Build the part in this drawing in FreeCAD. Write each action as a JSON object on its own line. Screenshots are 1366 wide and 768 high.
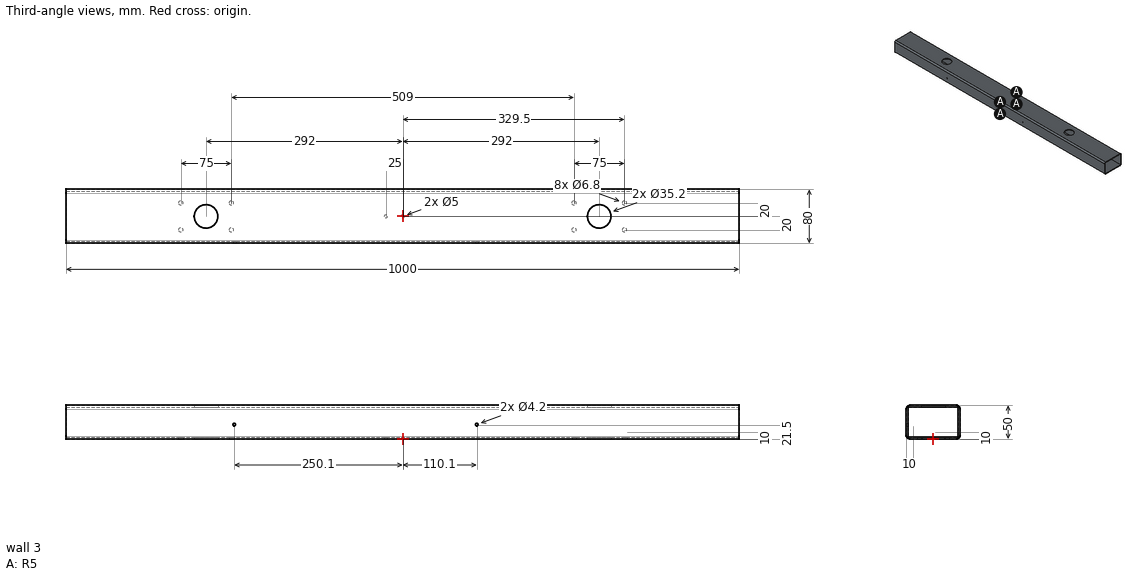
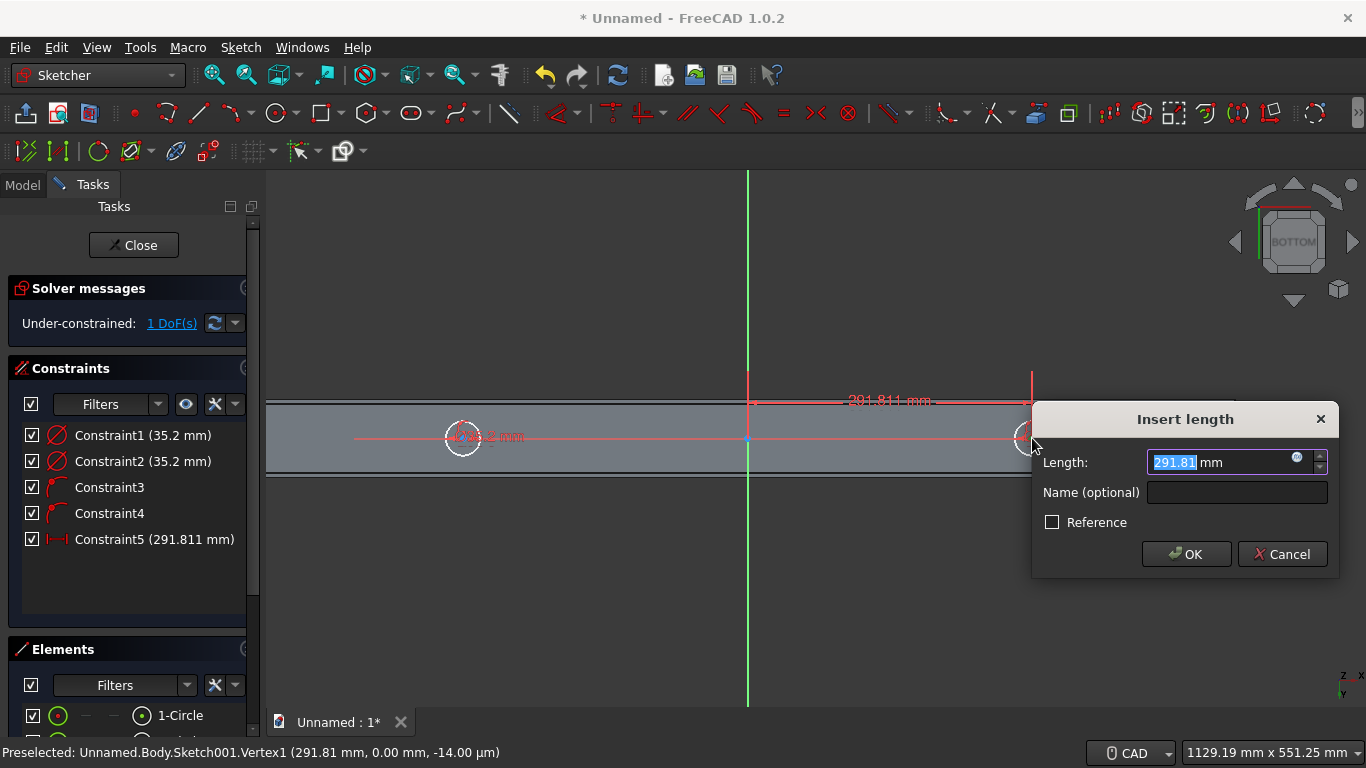
{"action": "type", "text": "292"}
{"action": "key", "text": "Return"}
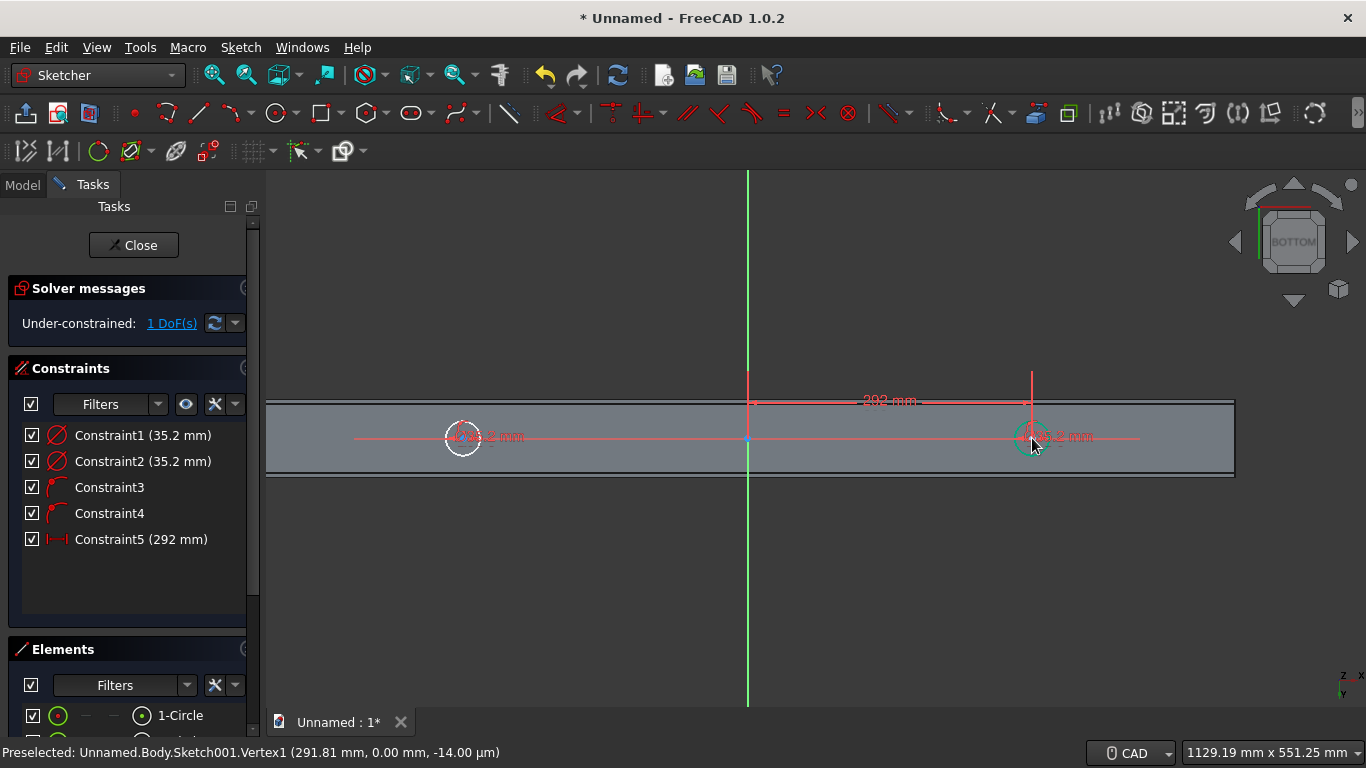
{"action": "left_click", "coordinate": [463, 438]}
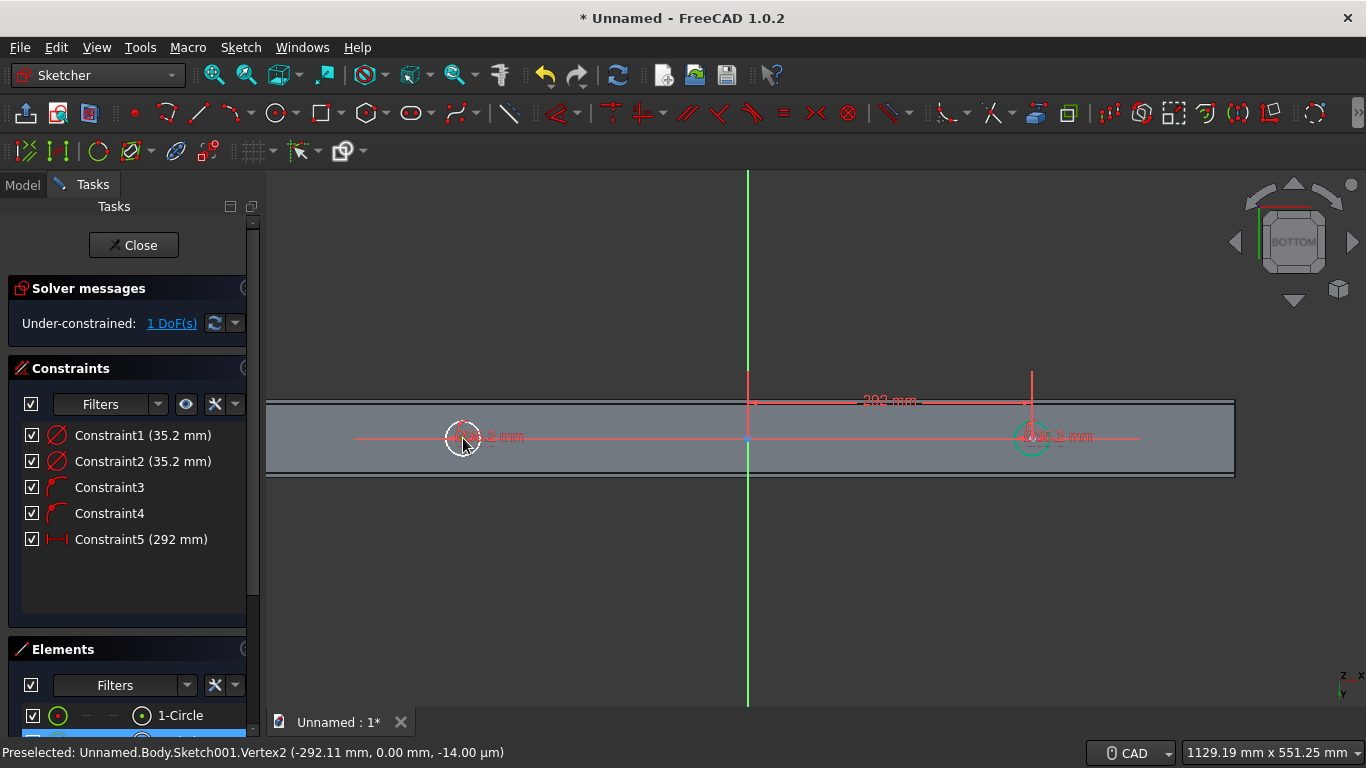
{"action": "key", "text": "l"}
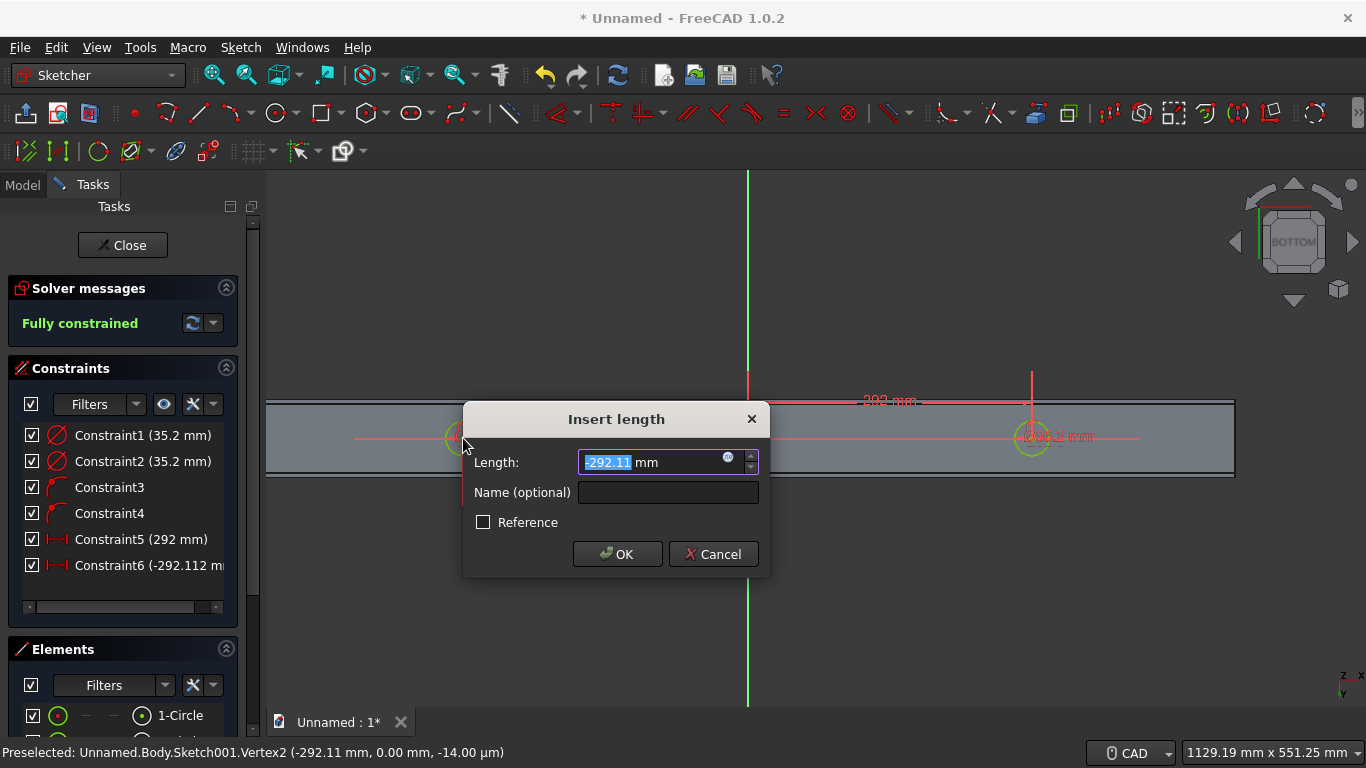
{"action": "type", "text": "-292"}
{"action": "key", "text": "Return"}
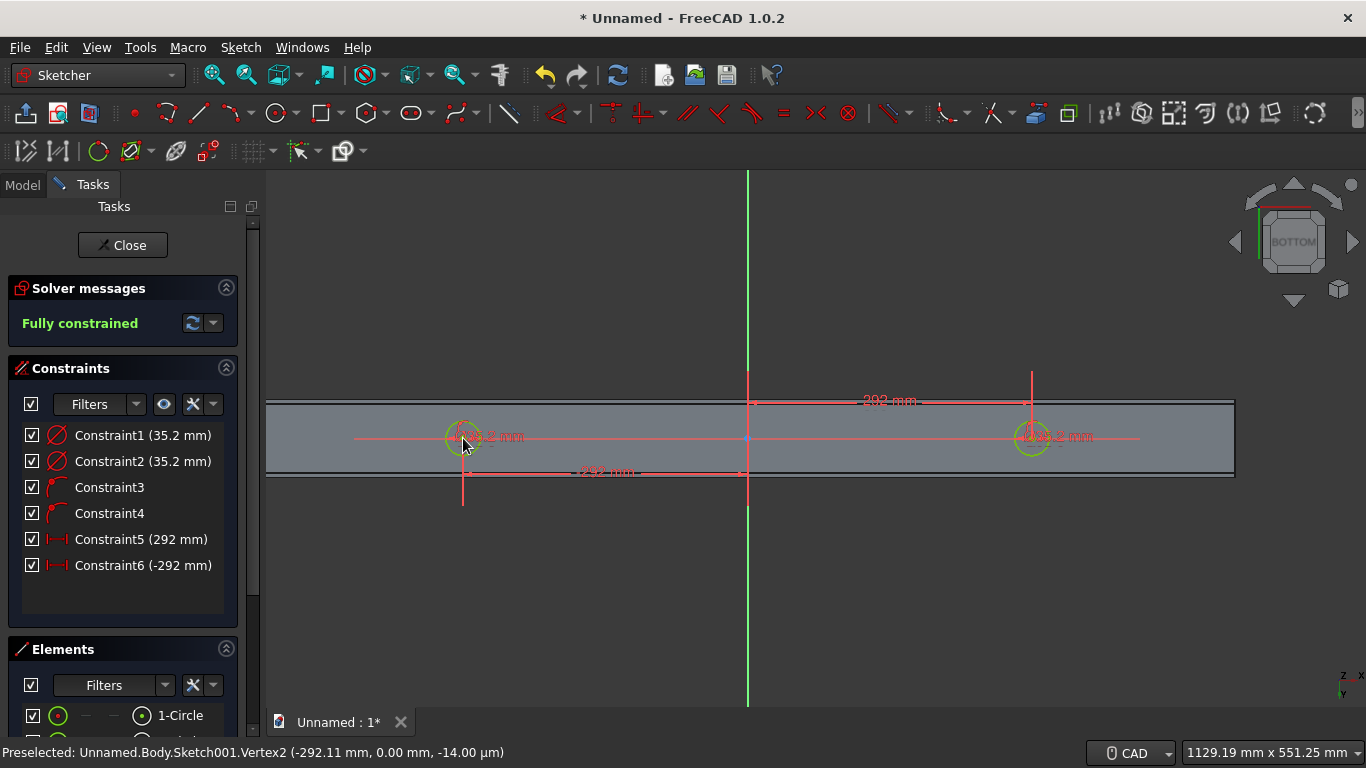
{"action": "left_click", "coordinate": [123, 245]}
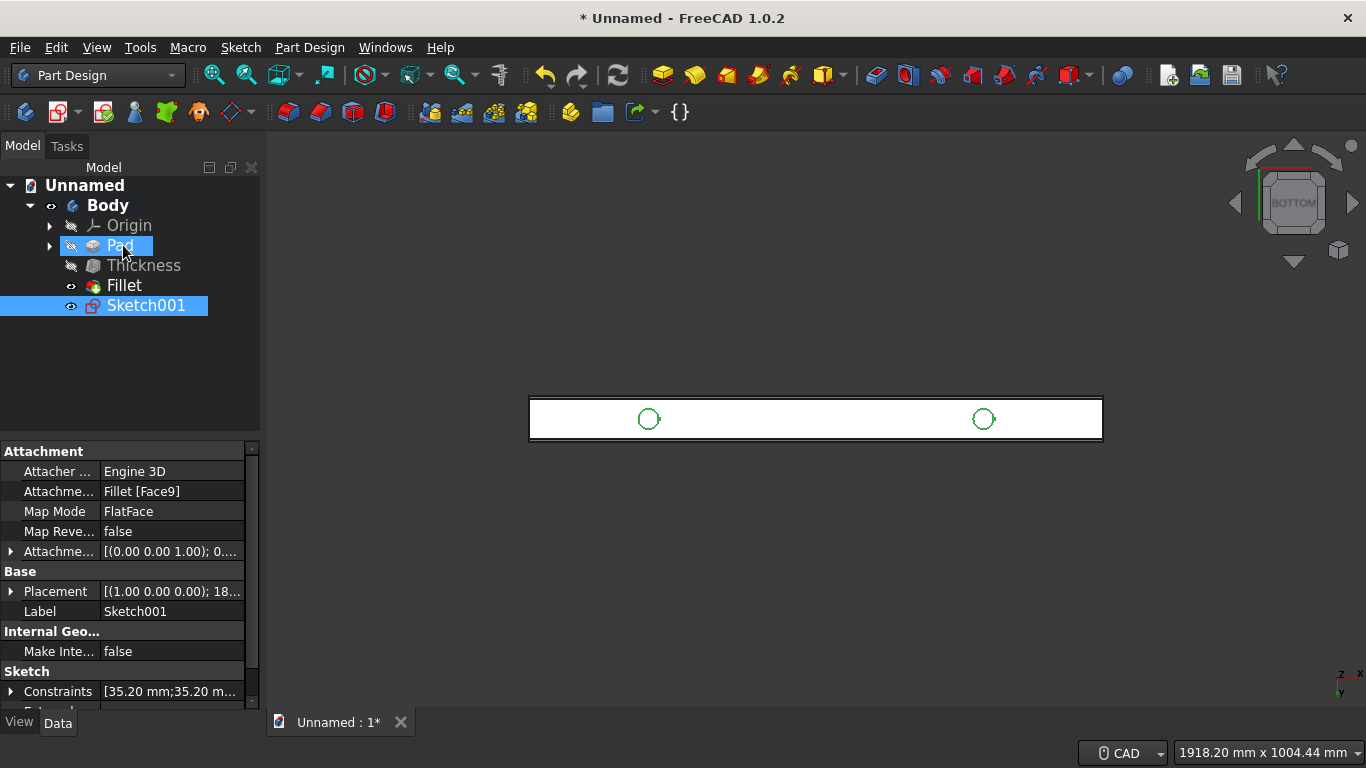
{"action": "left_click", "coordinate": [878, 76]}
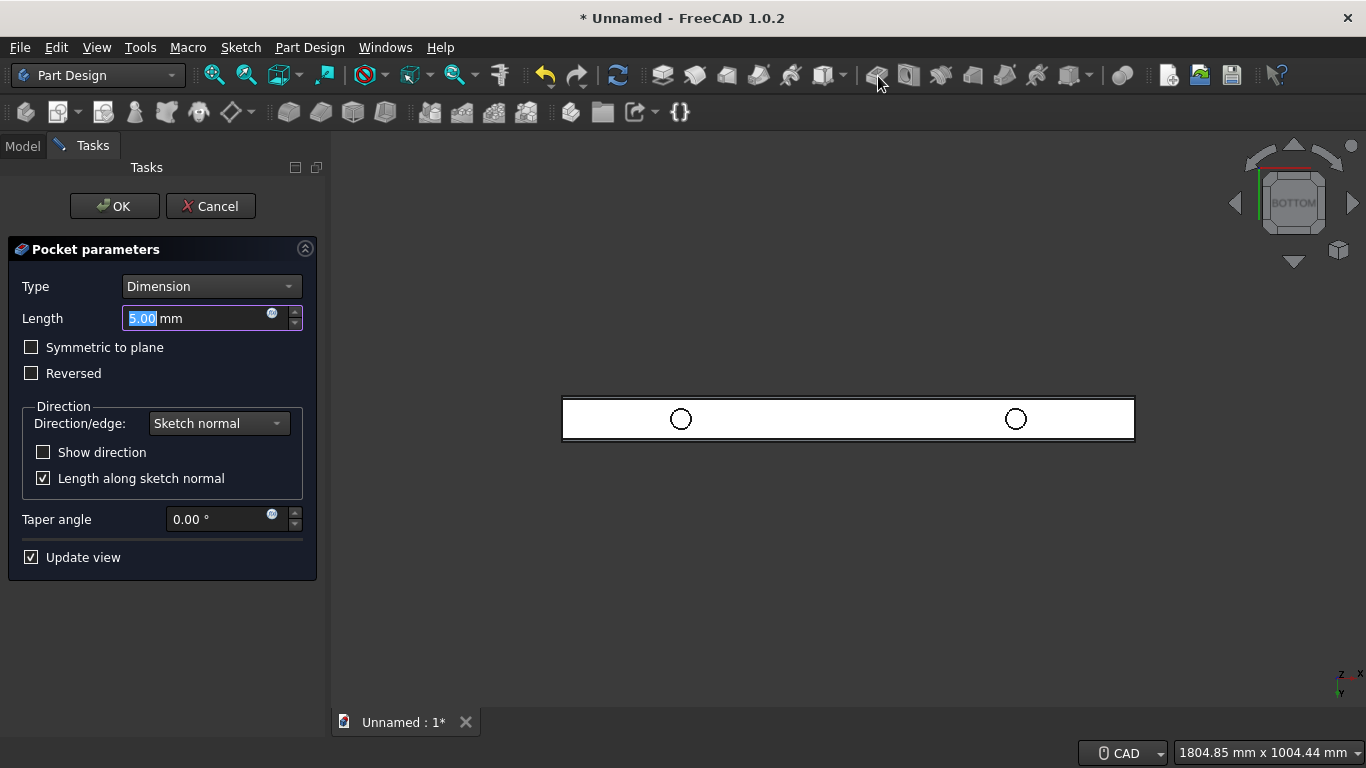
{"action": "left_click", "coordinate": [212, 286]}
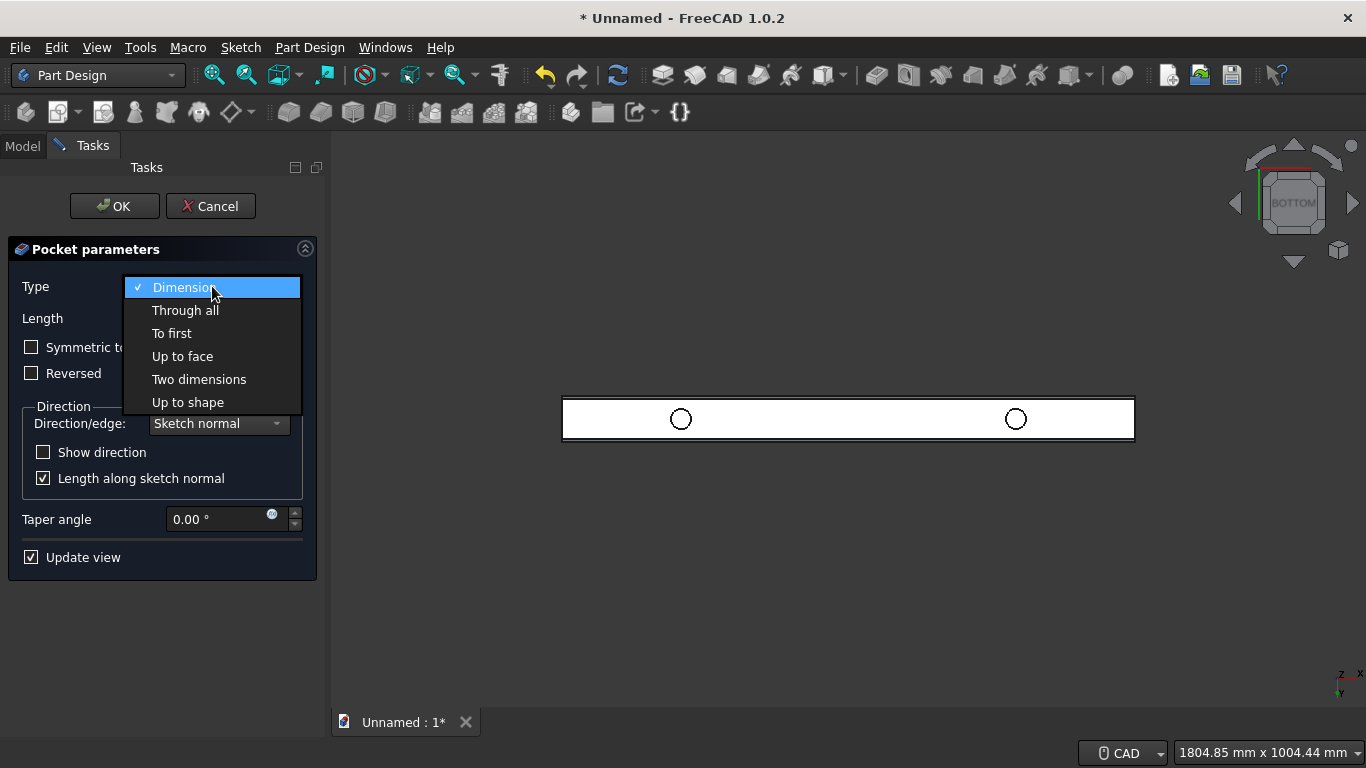
{"action": "left_click", "coordinate": [212, 310]}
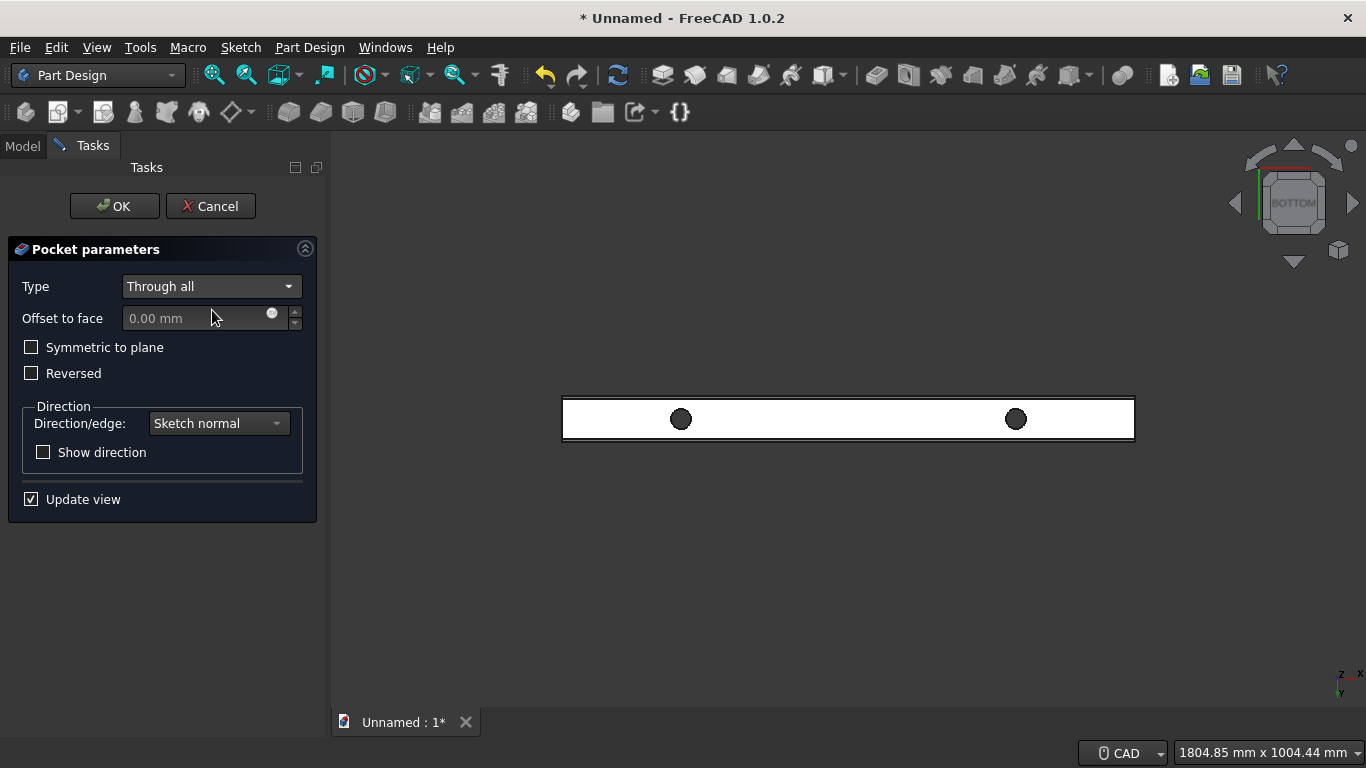
{"action": "left_click", "coordinate": [115, 206]}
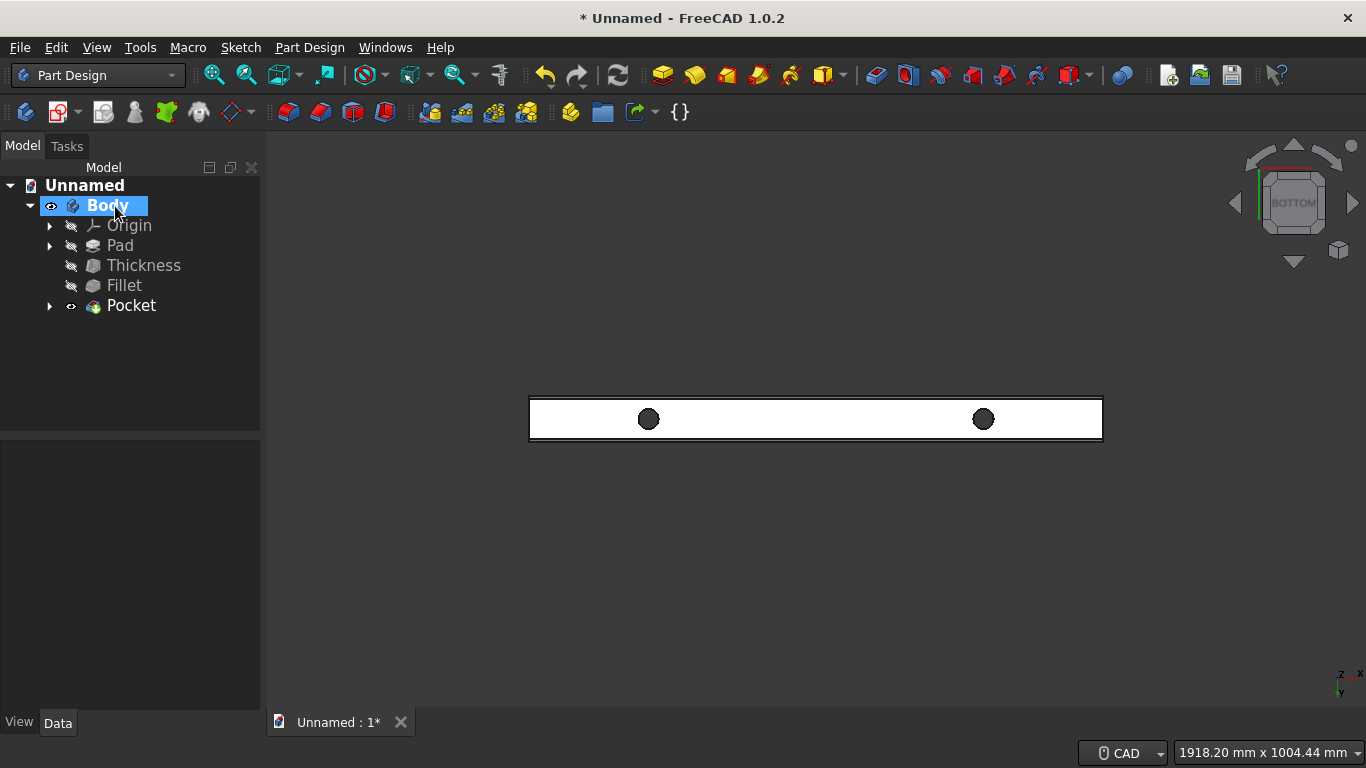
{"action": "left_click", "coordinate": [58, 112]}